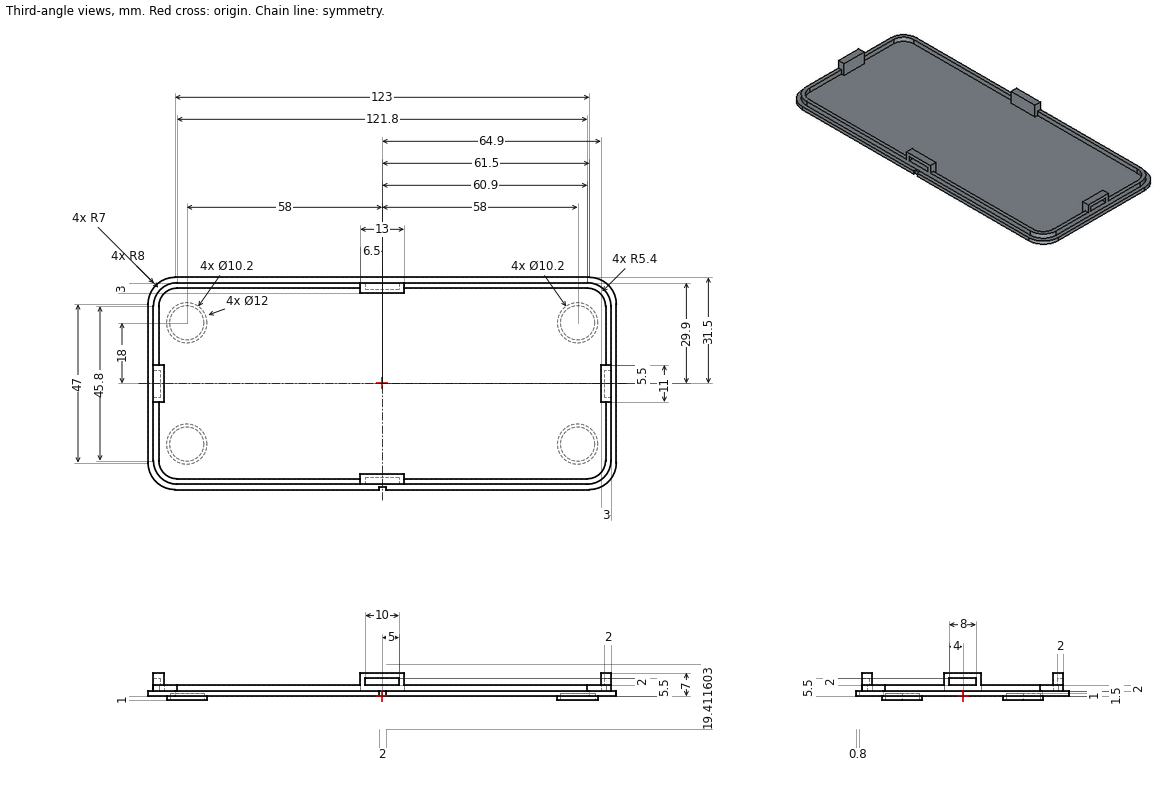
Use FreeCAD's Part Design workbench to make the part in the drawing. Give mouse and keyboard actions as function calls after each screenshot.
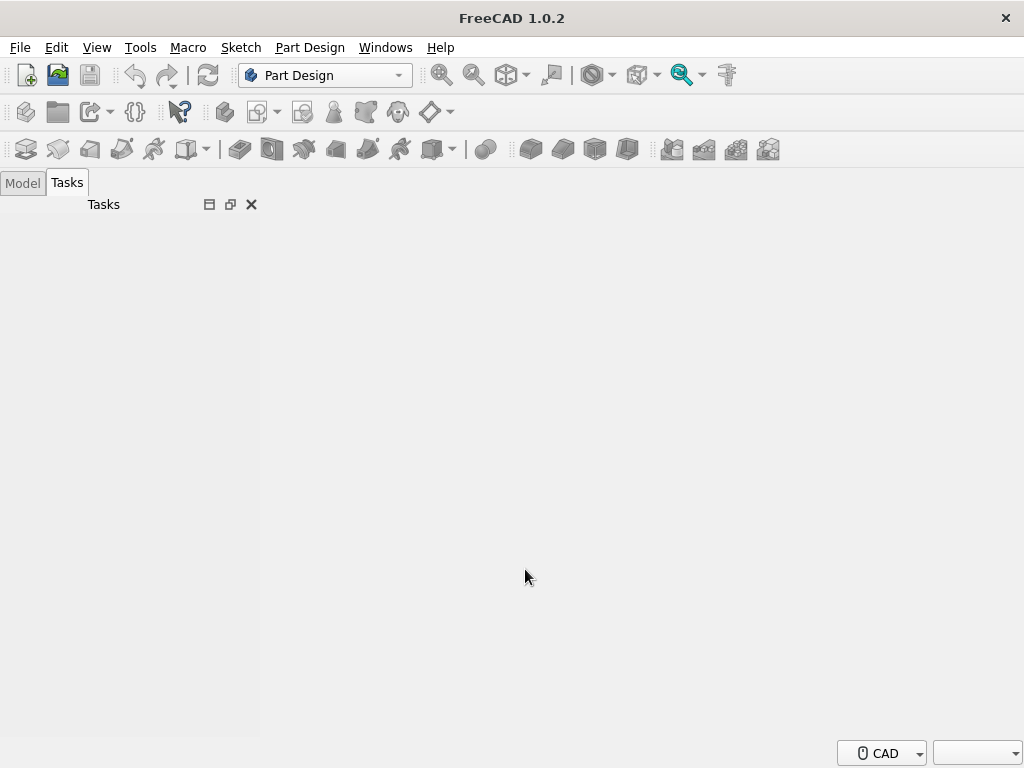
click(26, 76)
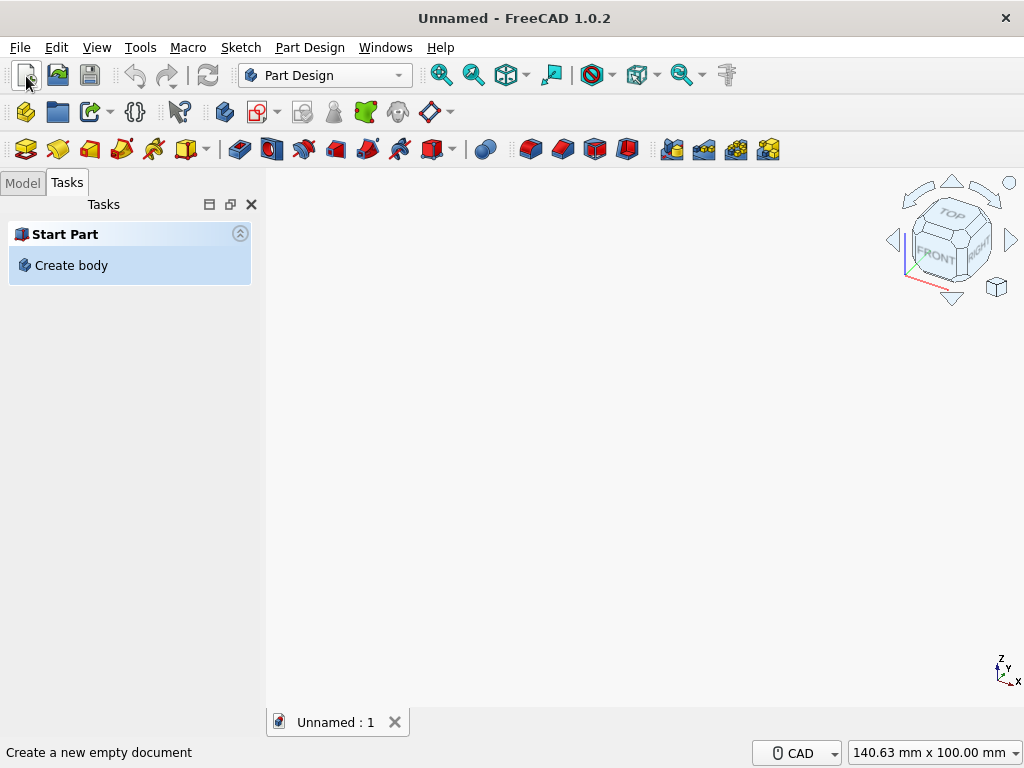
click(258, 112)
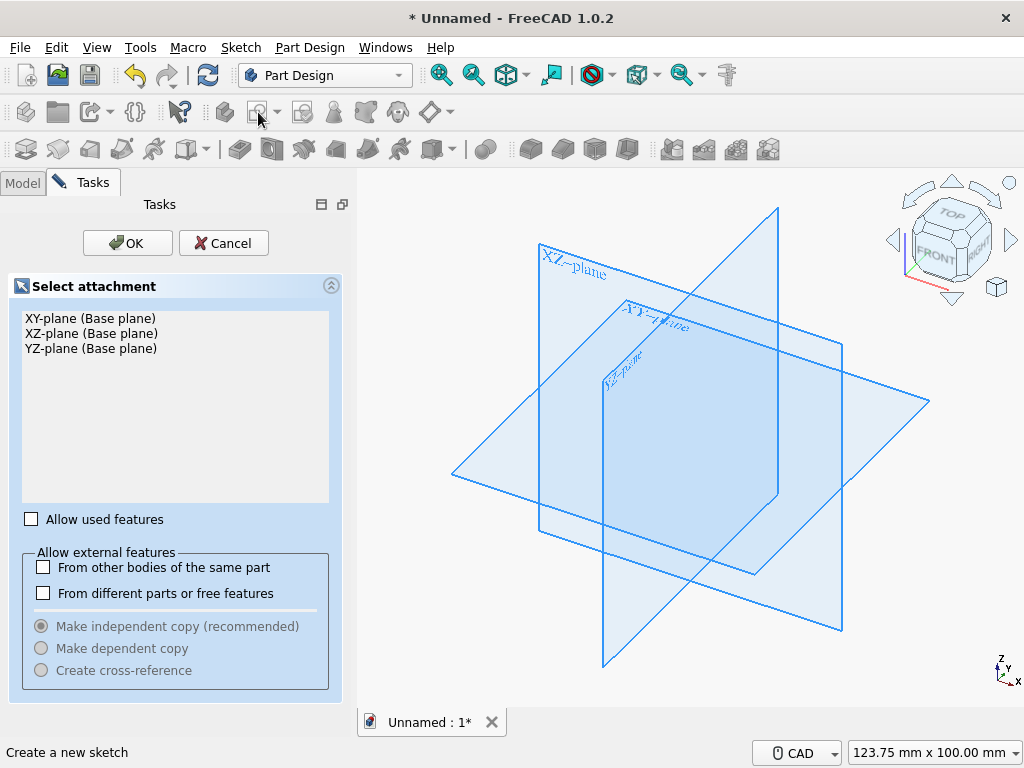
click(82, 318)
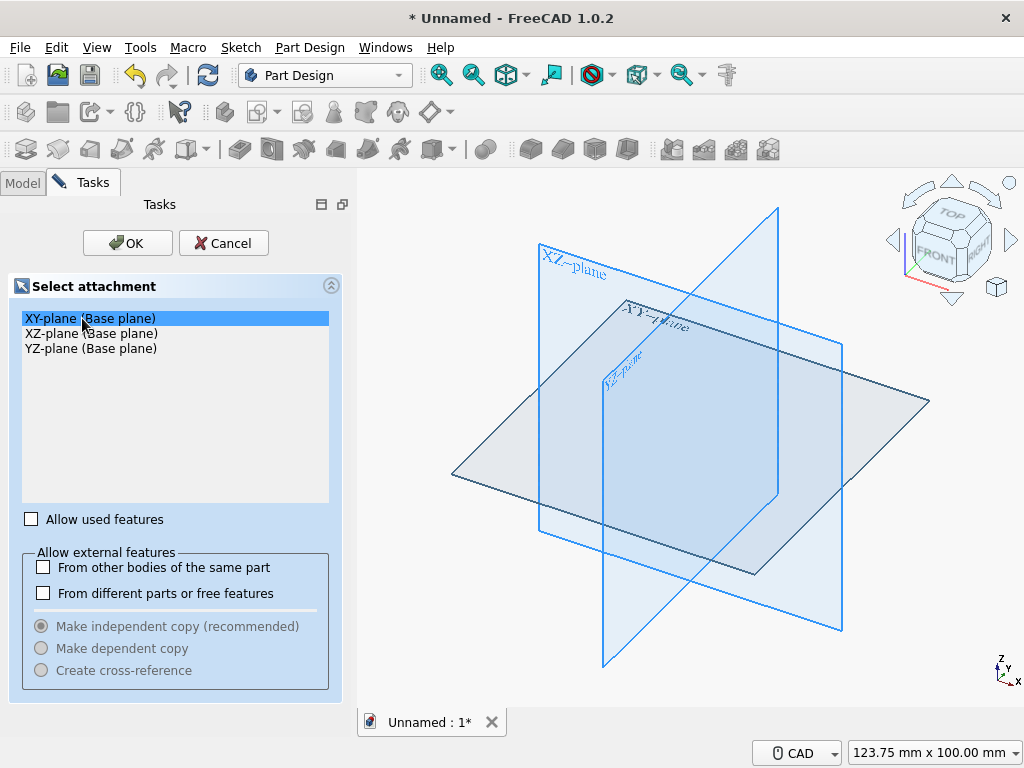
click(128, 243)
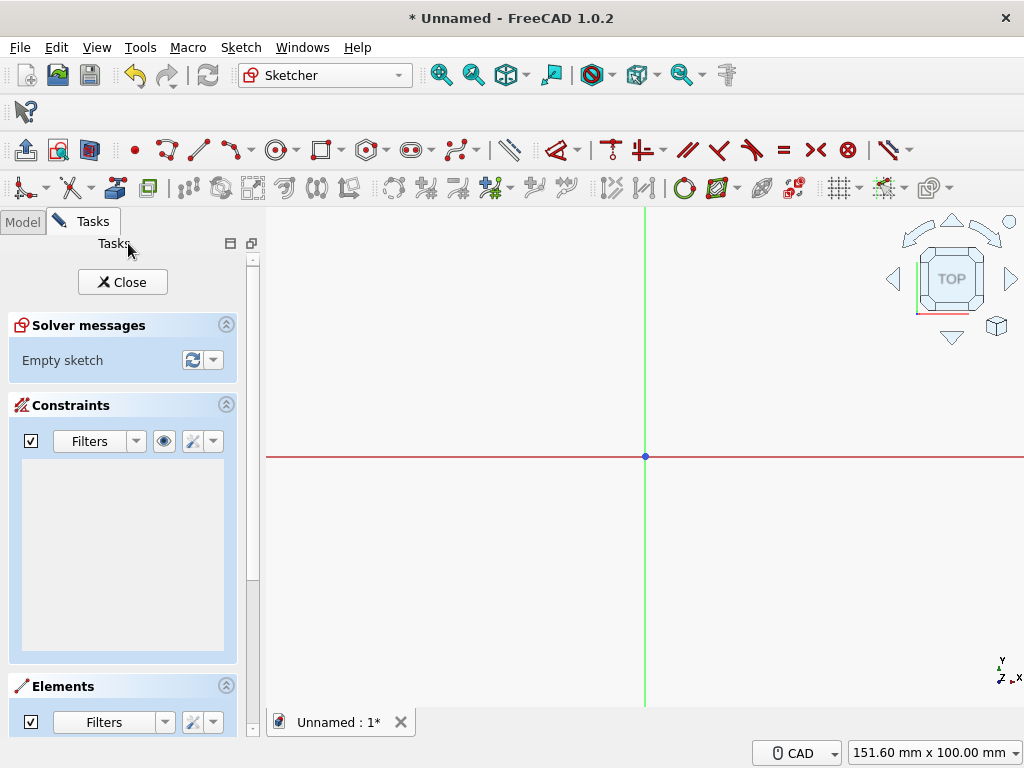
scroll(493, 457, down, 3)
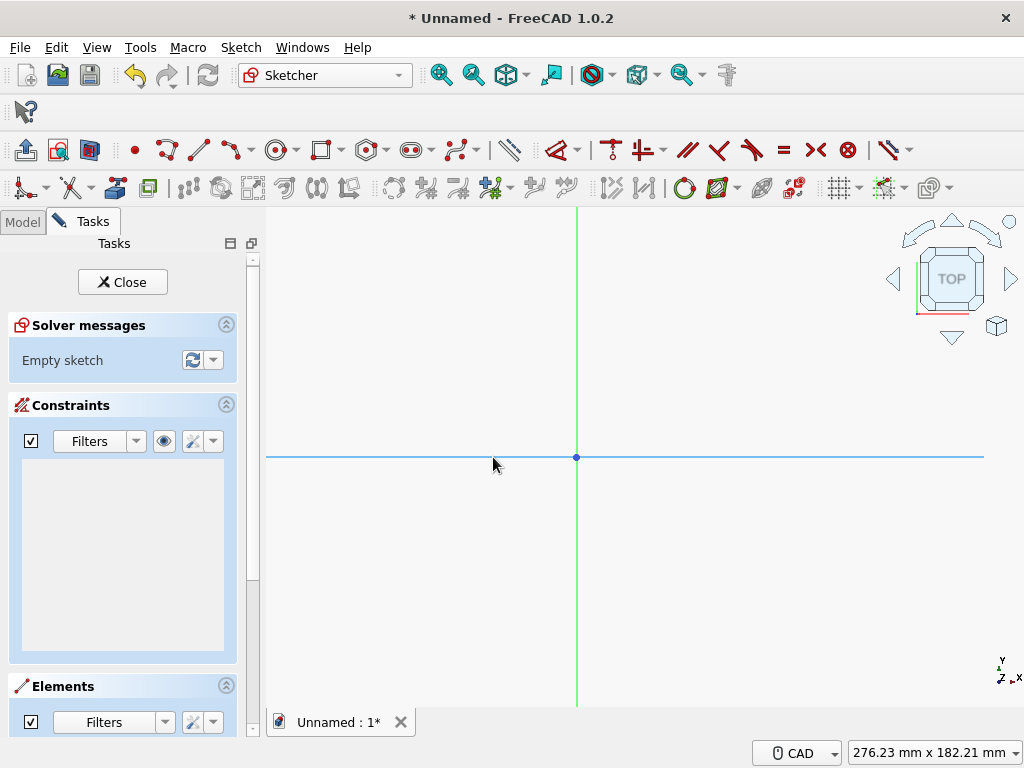
key(g)
key(l)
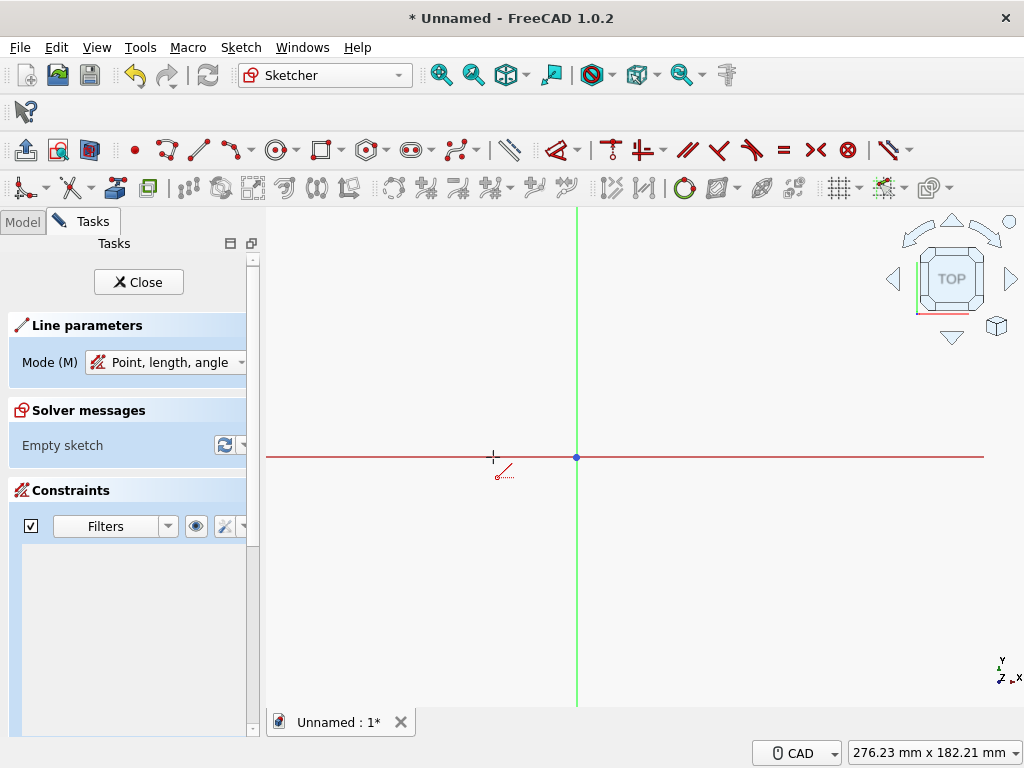
click(745, 371)
click(408, 371)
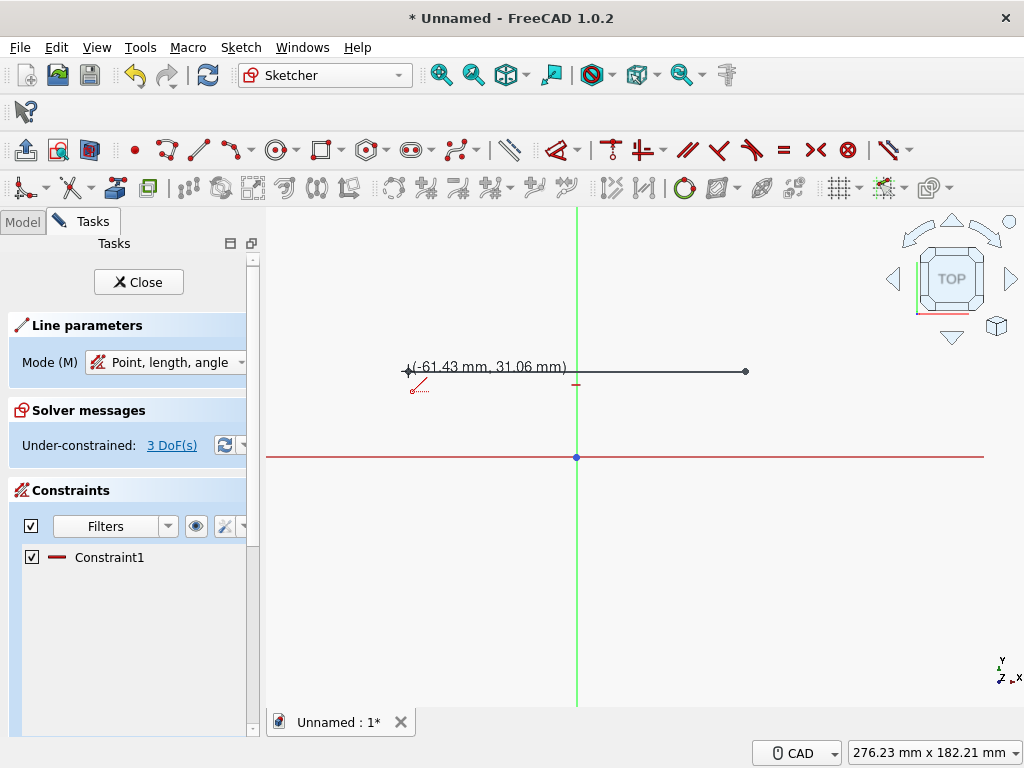
click(386, 393)
click(386, 522)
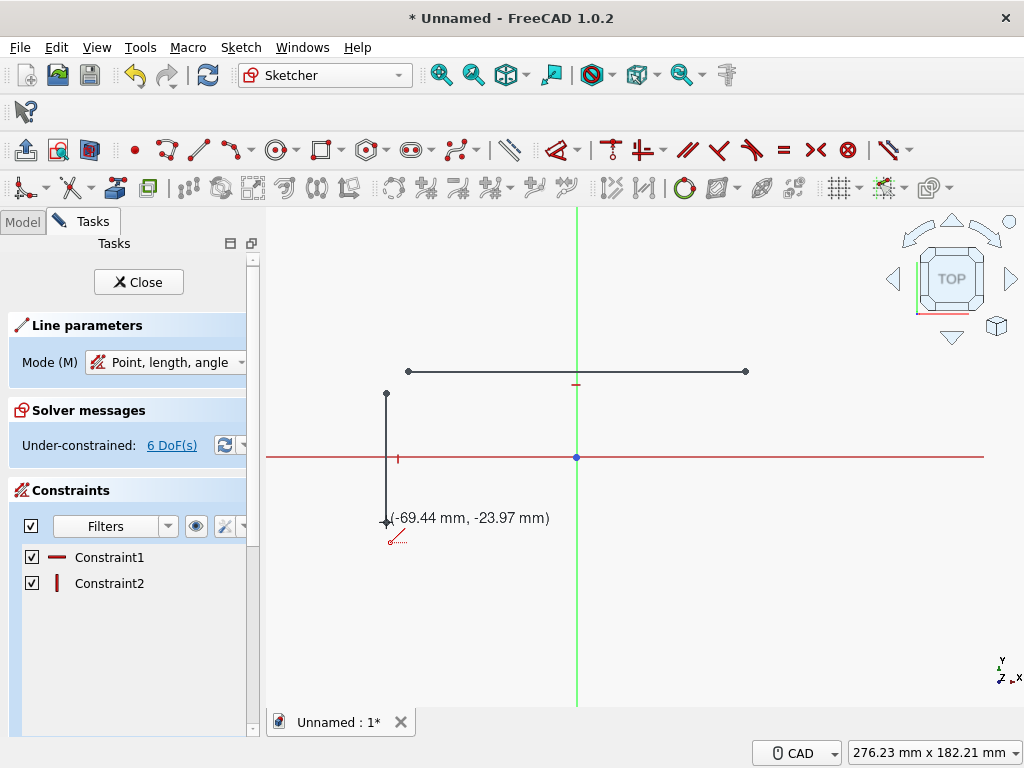
click(408, 544)
click(745, 544)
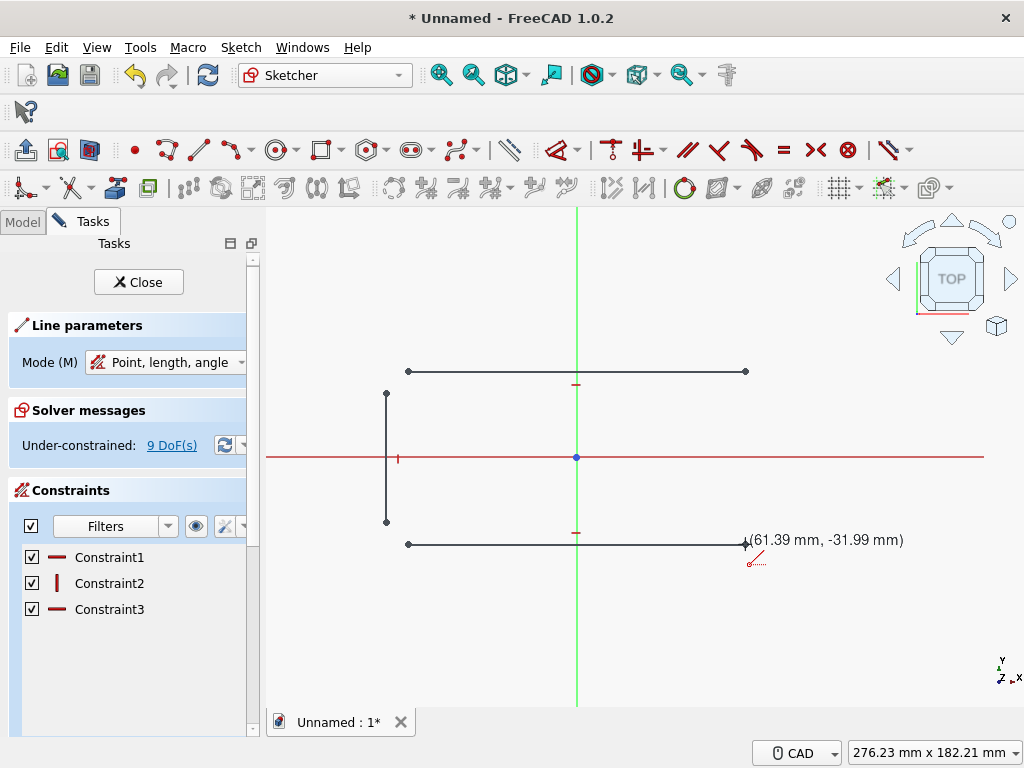
click(767, 522)
click(767, 393)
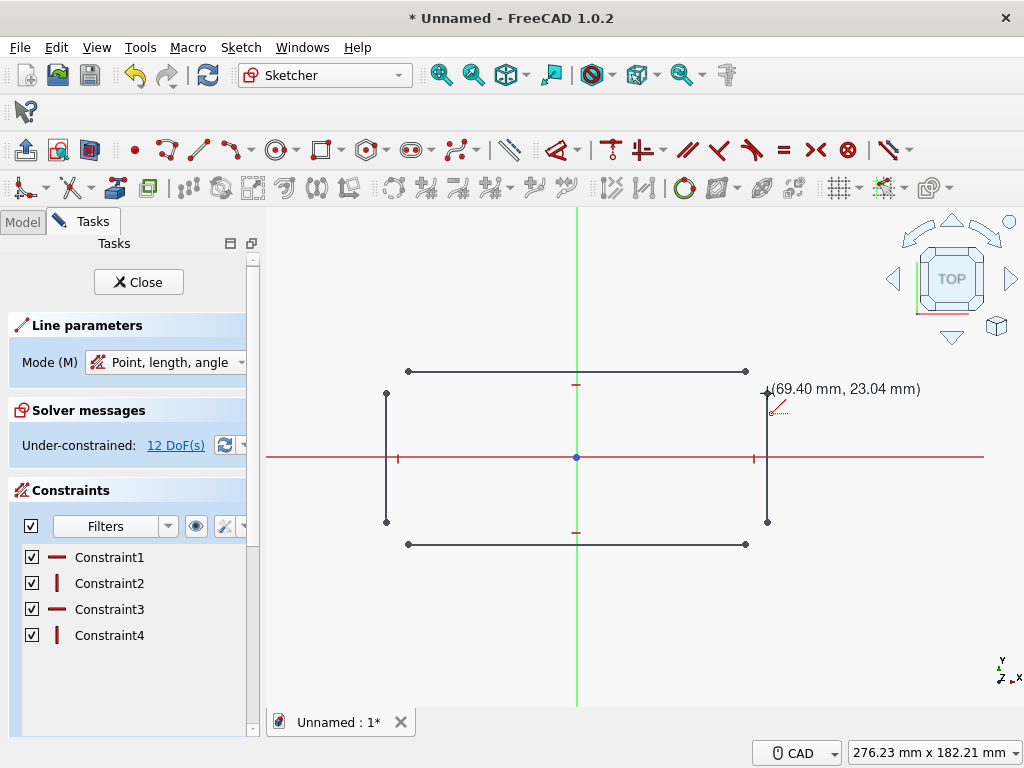
key(g)
key(3)
key(a)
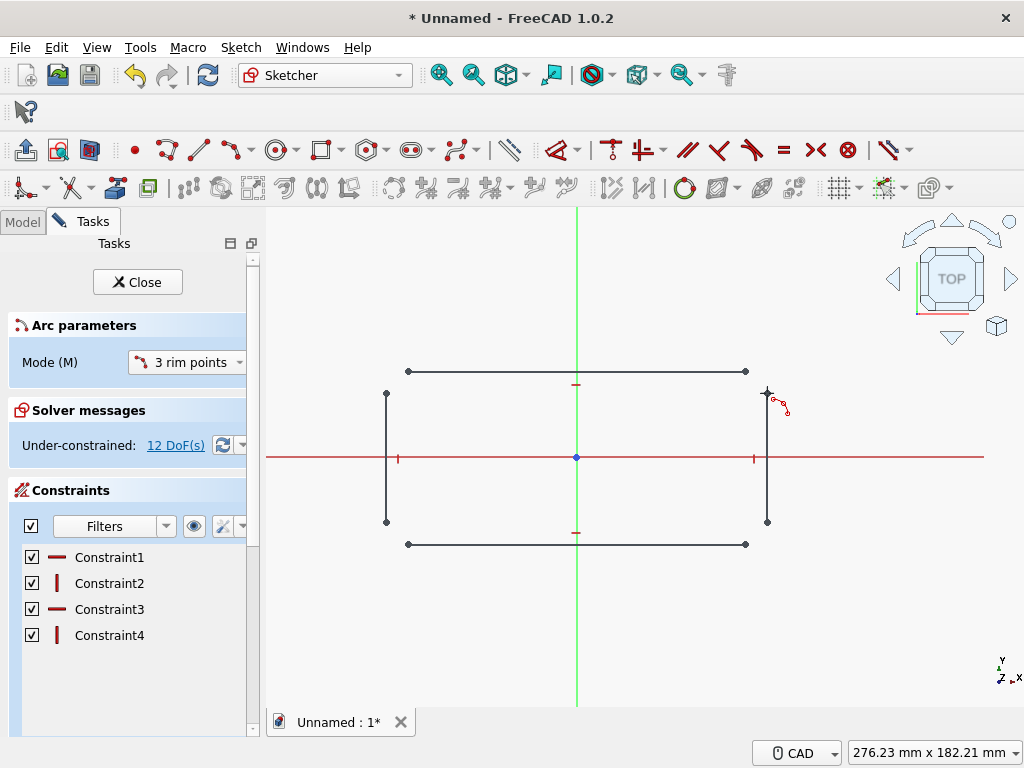
click(408, 372)
click(386, 394)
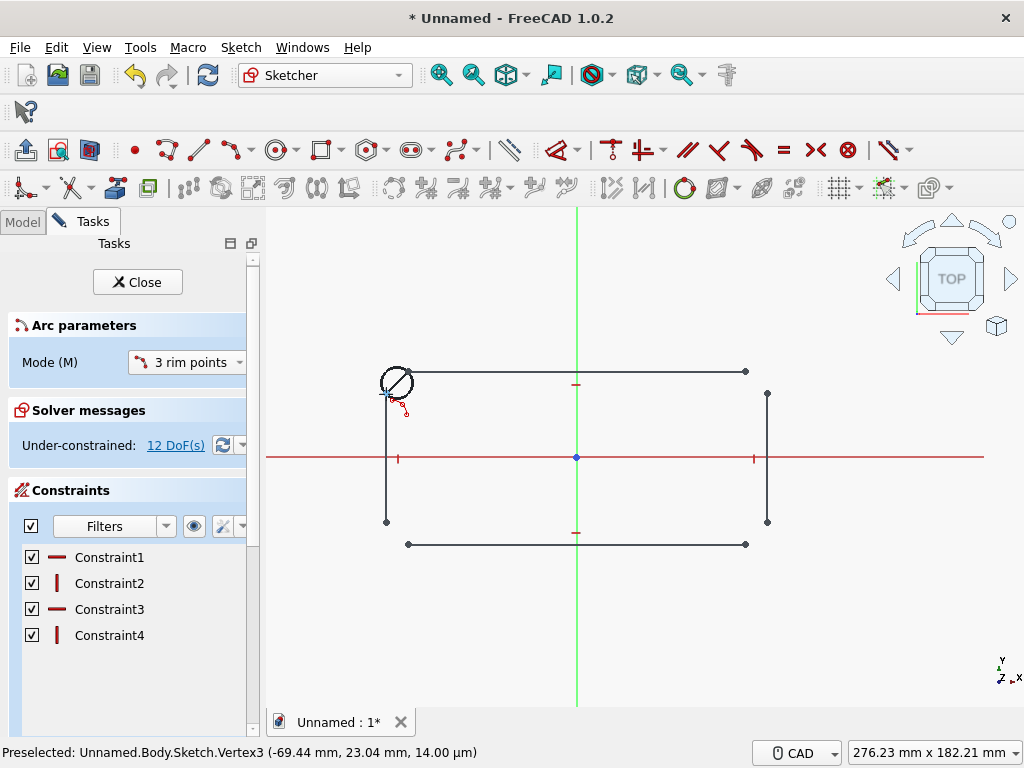
scroll(392, 377, up, 5)